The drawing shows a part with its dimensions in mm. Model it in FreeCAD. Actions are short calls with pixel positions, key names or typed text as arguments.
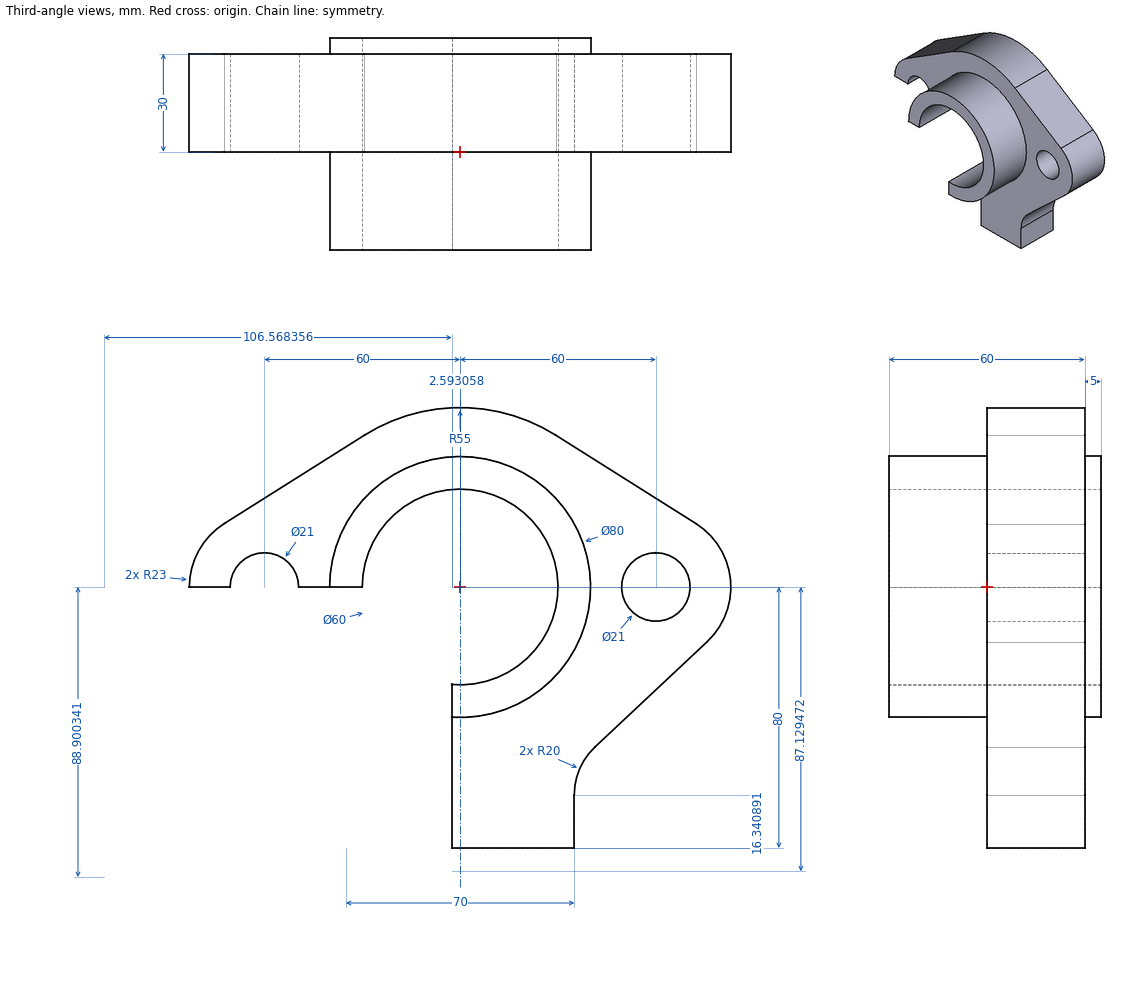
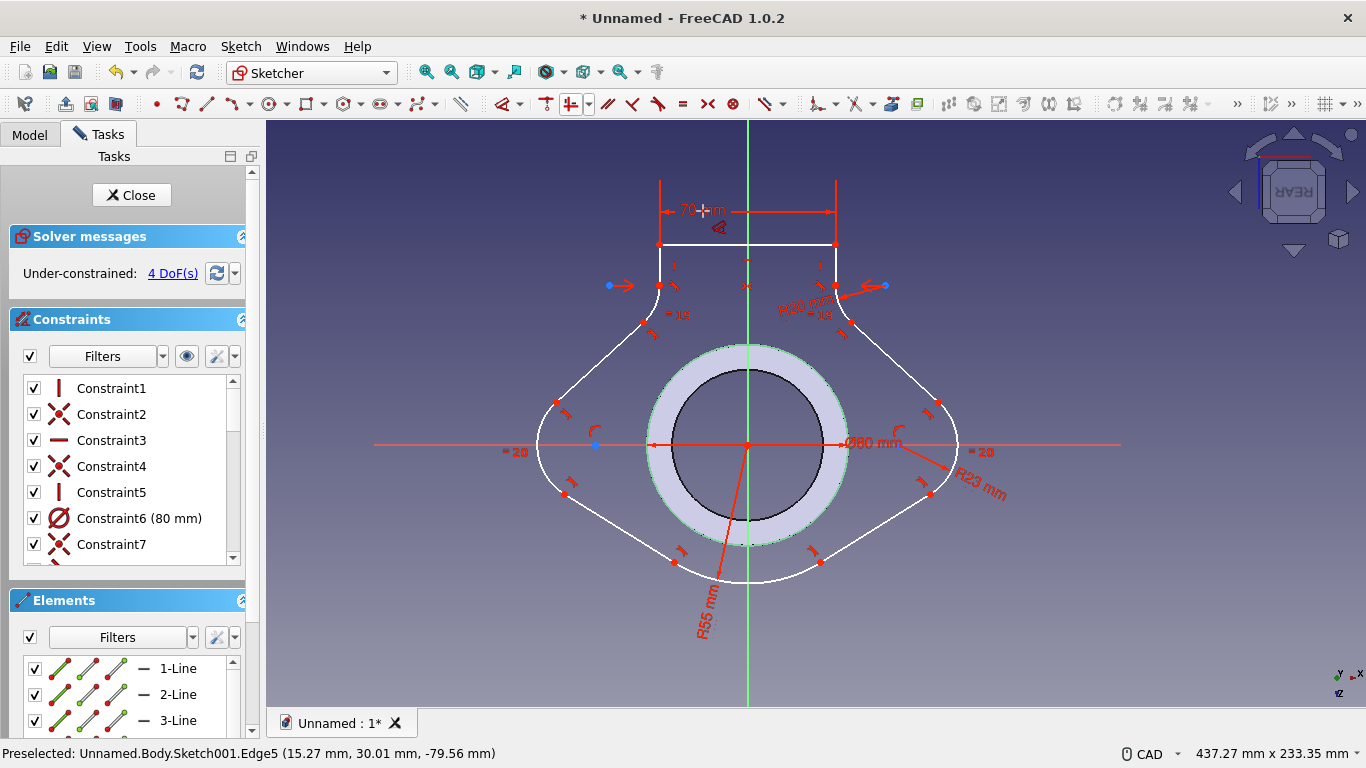
click(836, 245)
click(870, 391)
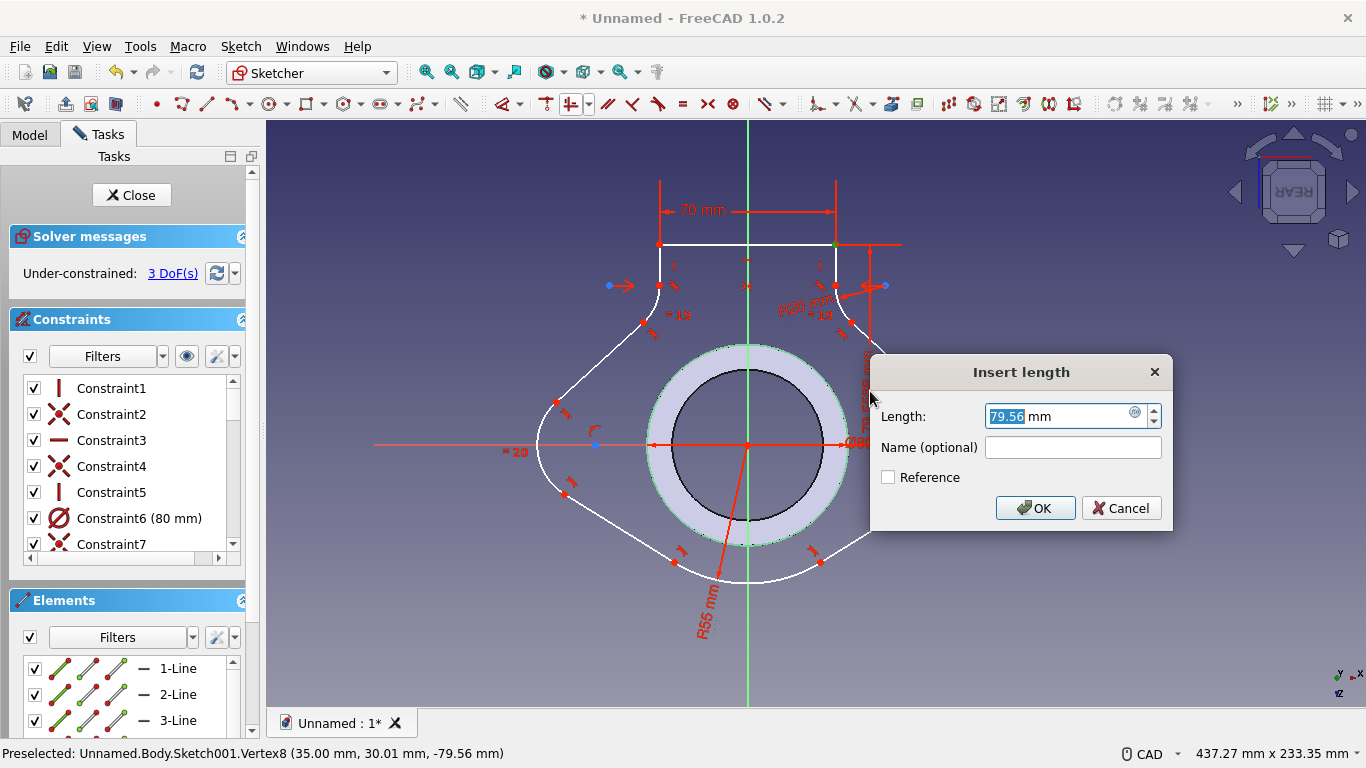
text(80)
key(Return)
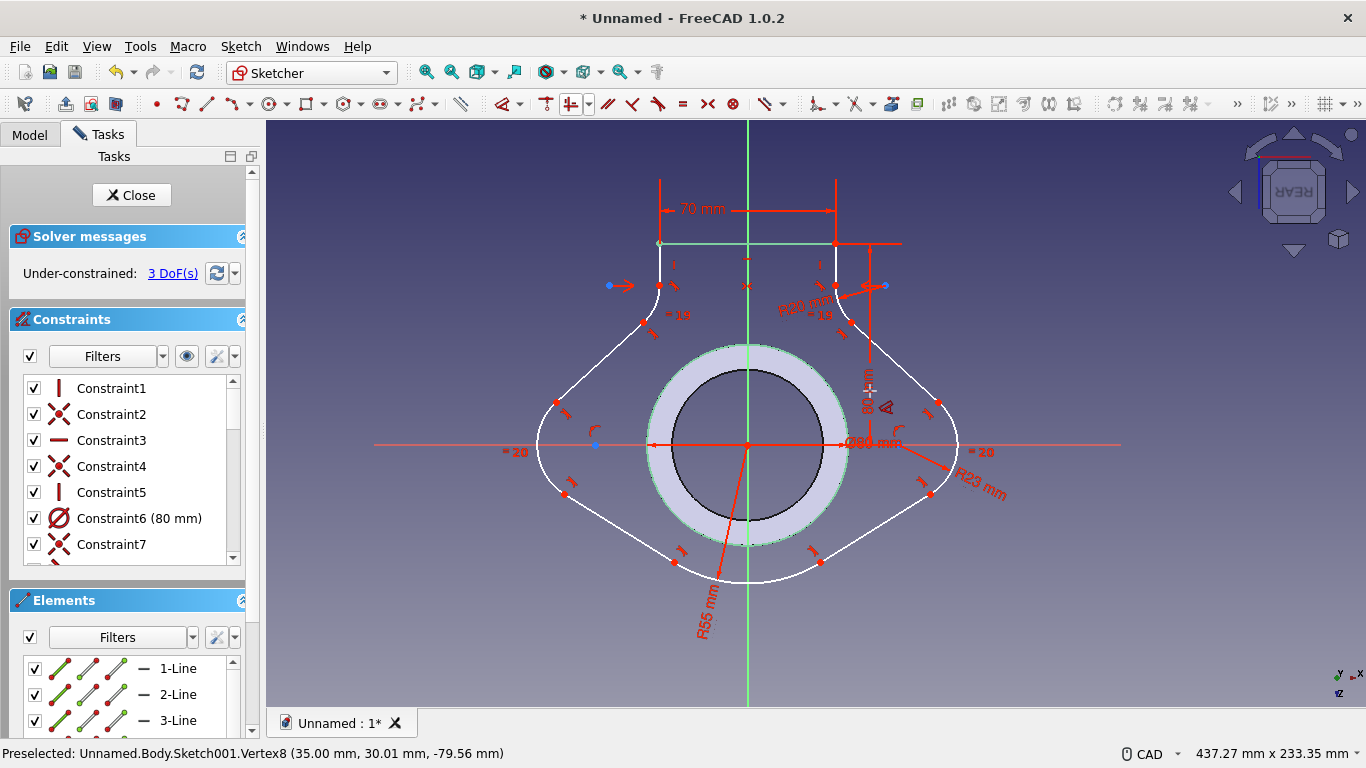
click(900, 445)
click(824, 479)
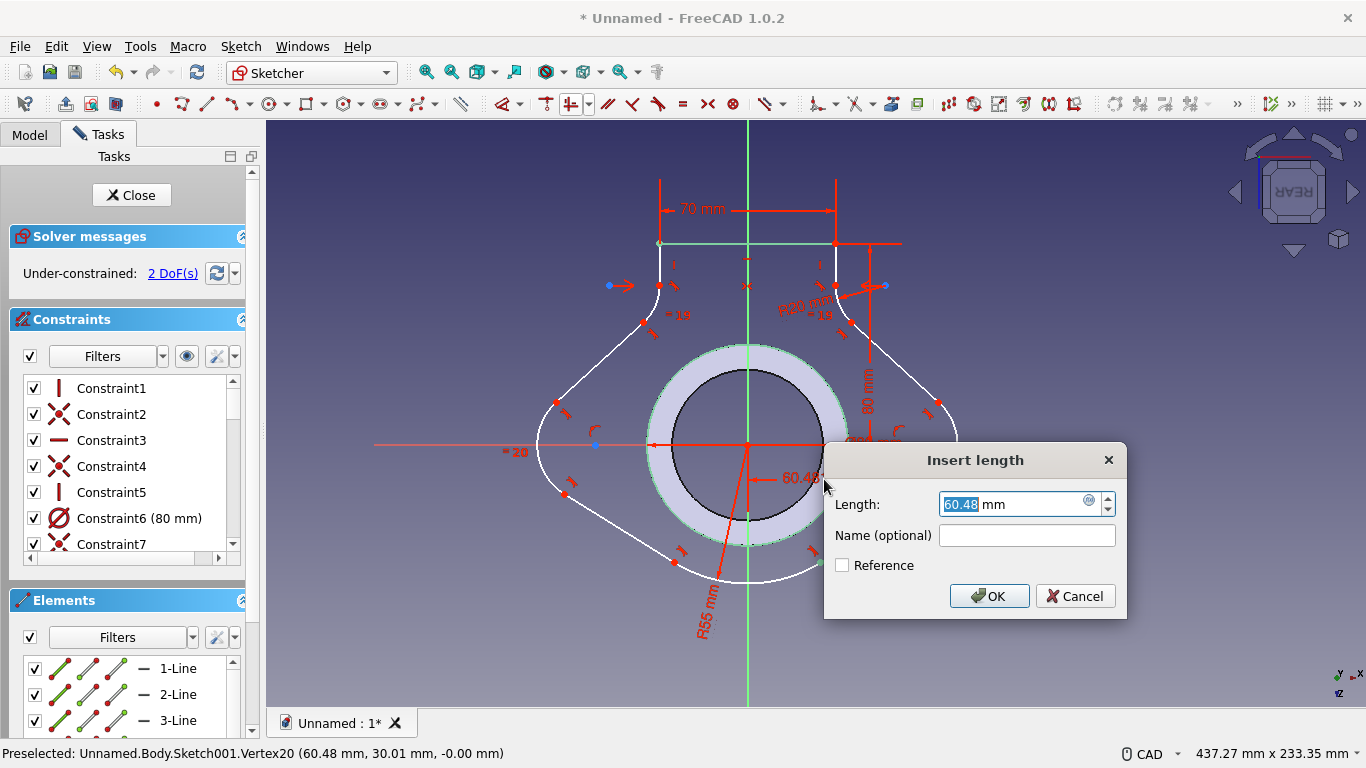
text(60)
key(Return)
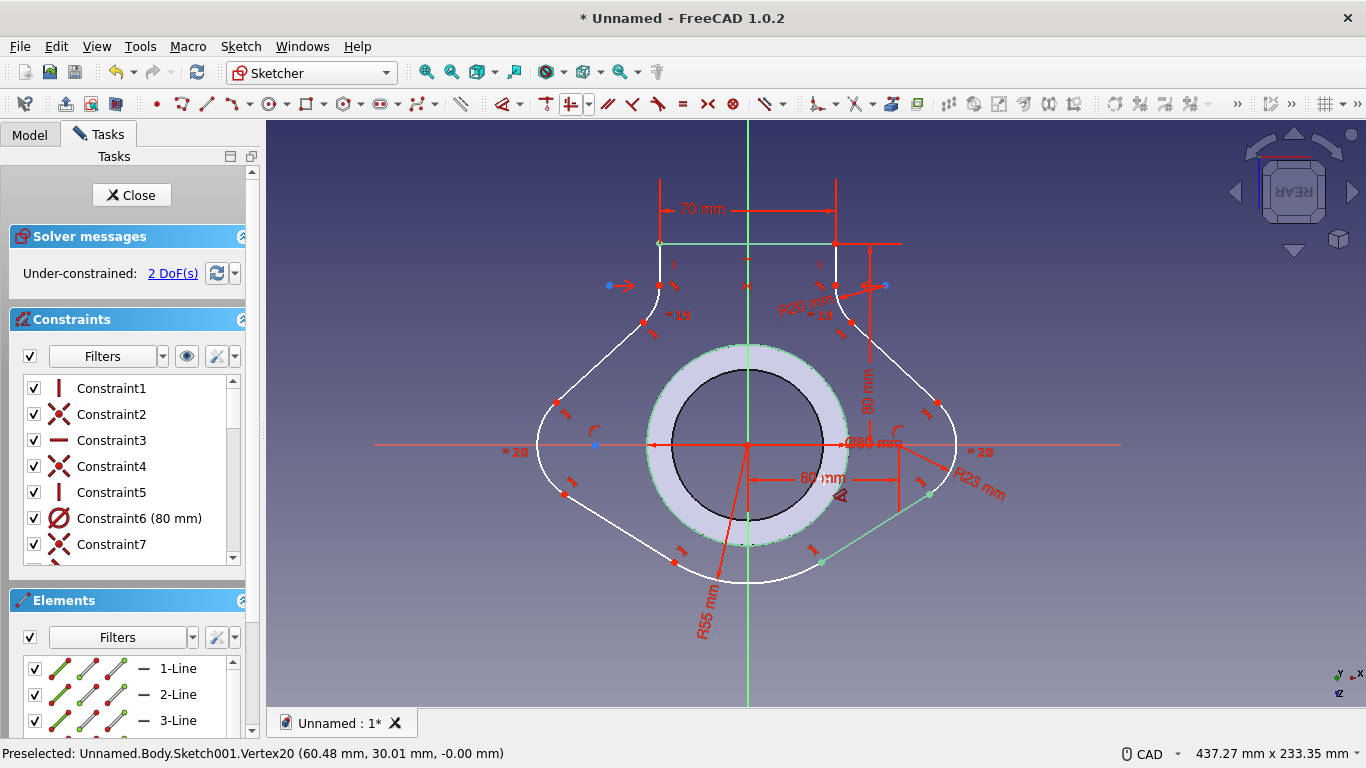
click(595, 445)
click(671, 479)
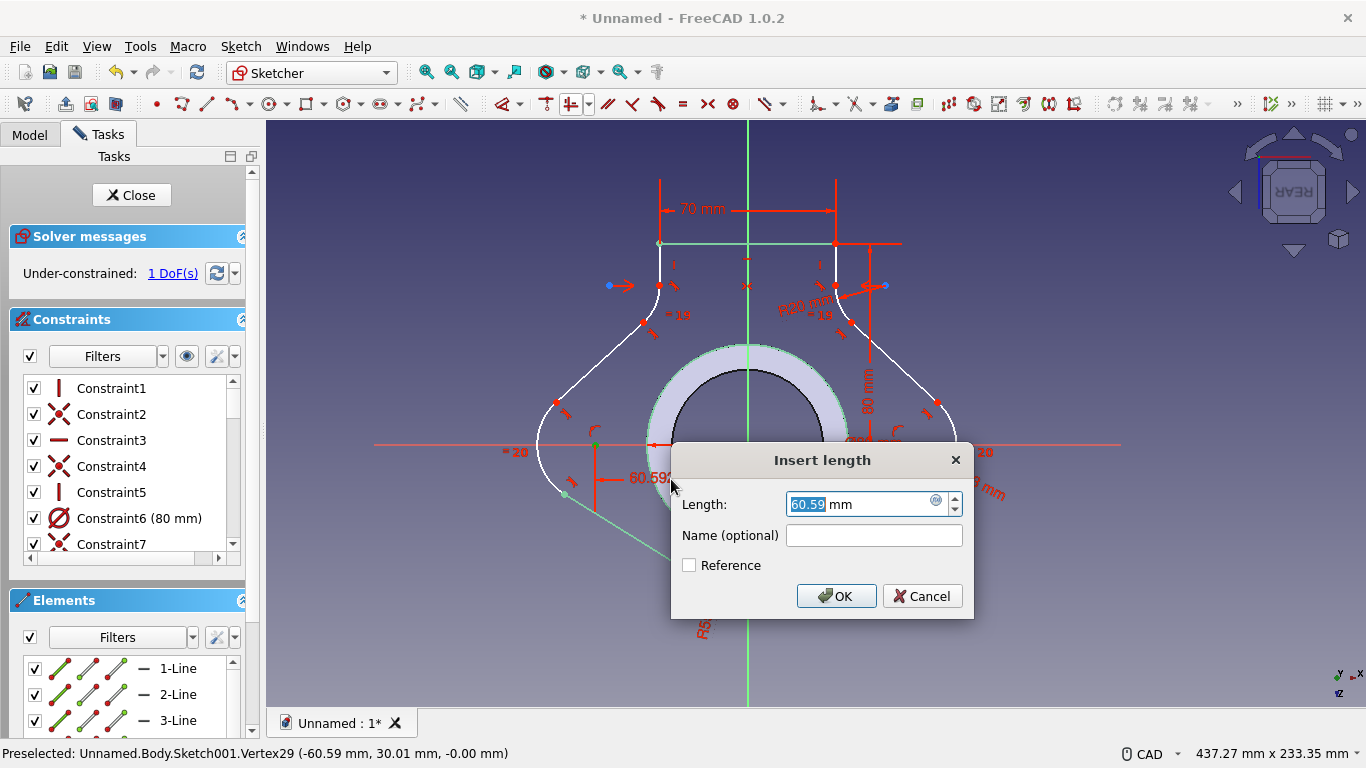
text(60)
key(Return)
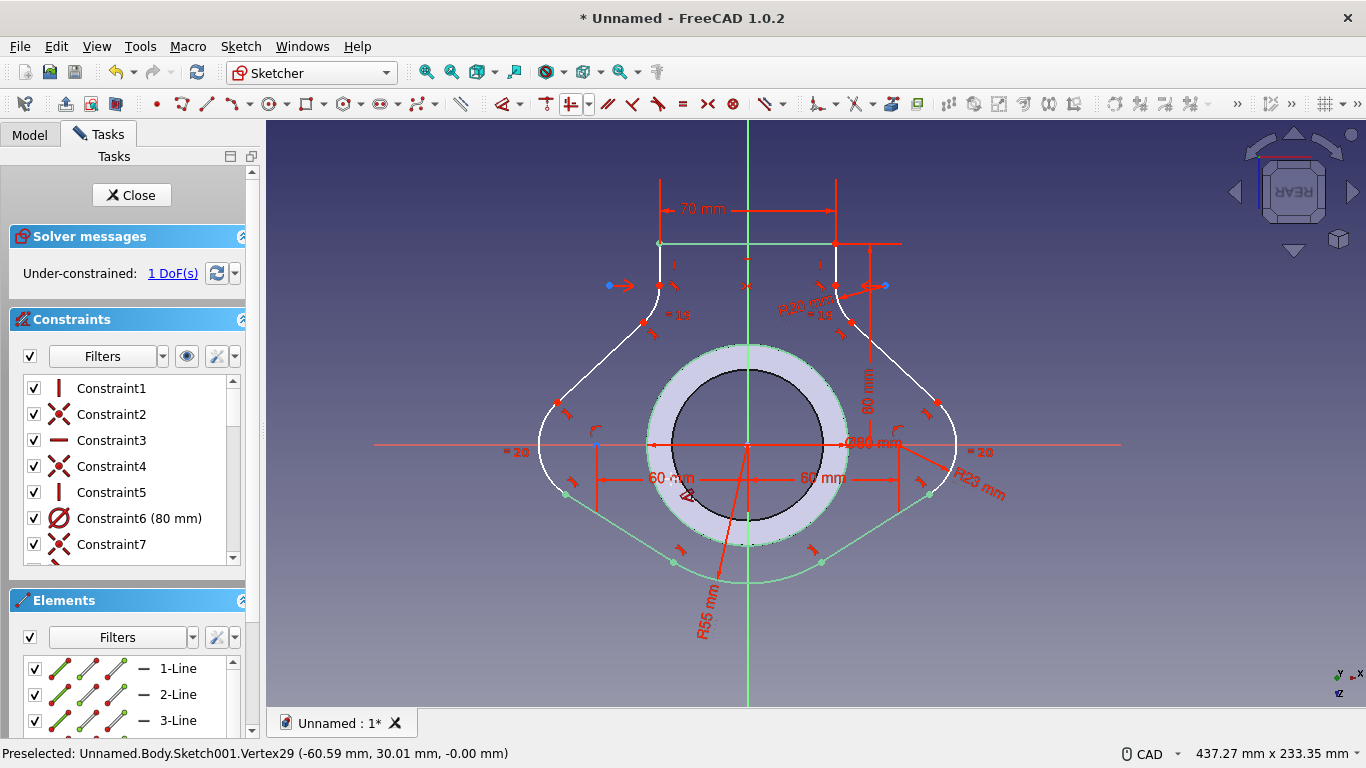
click(836, 273)
click(870, 265)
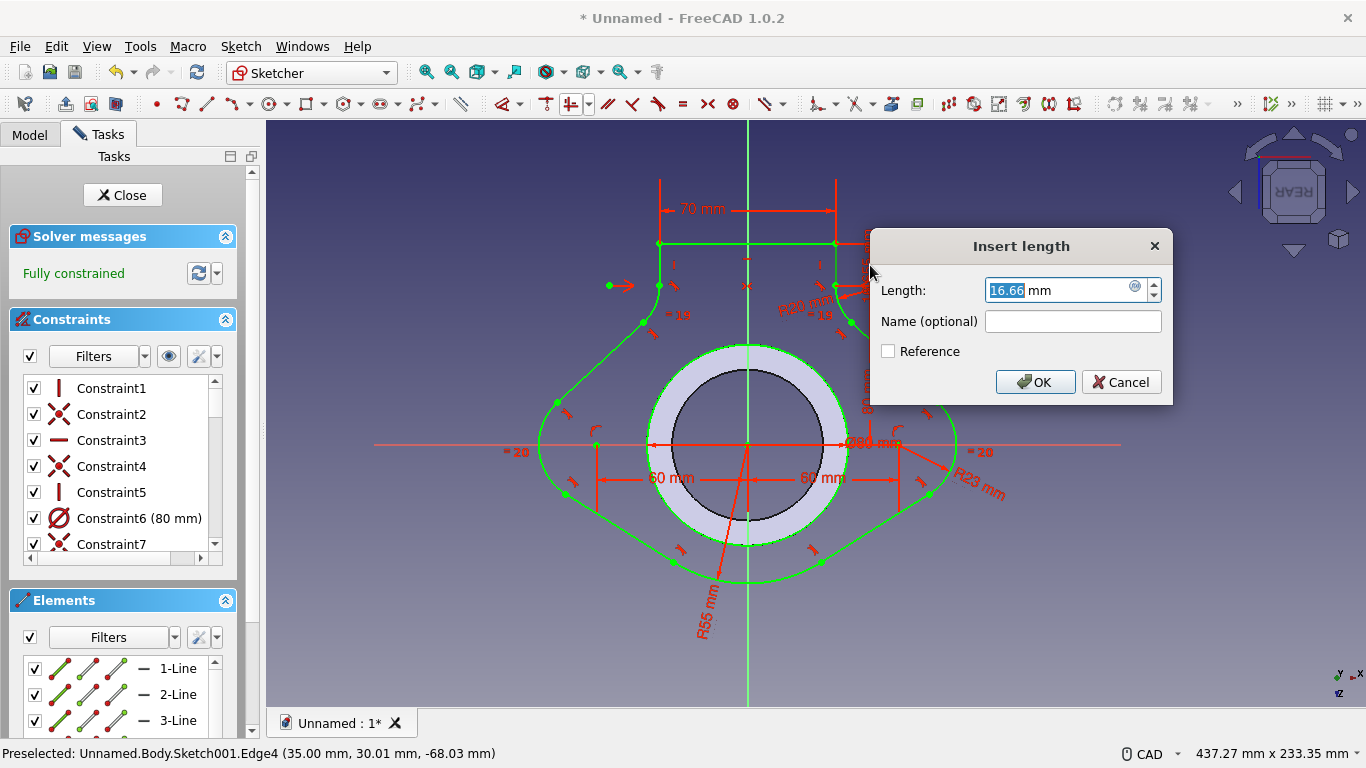
text(16.340891)
key(Return)
key(Escape)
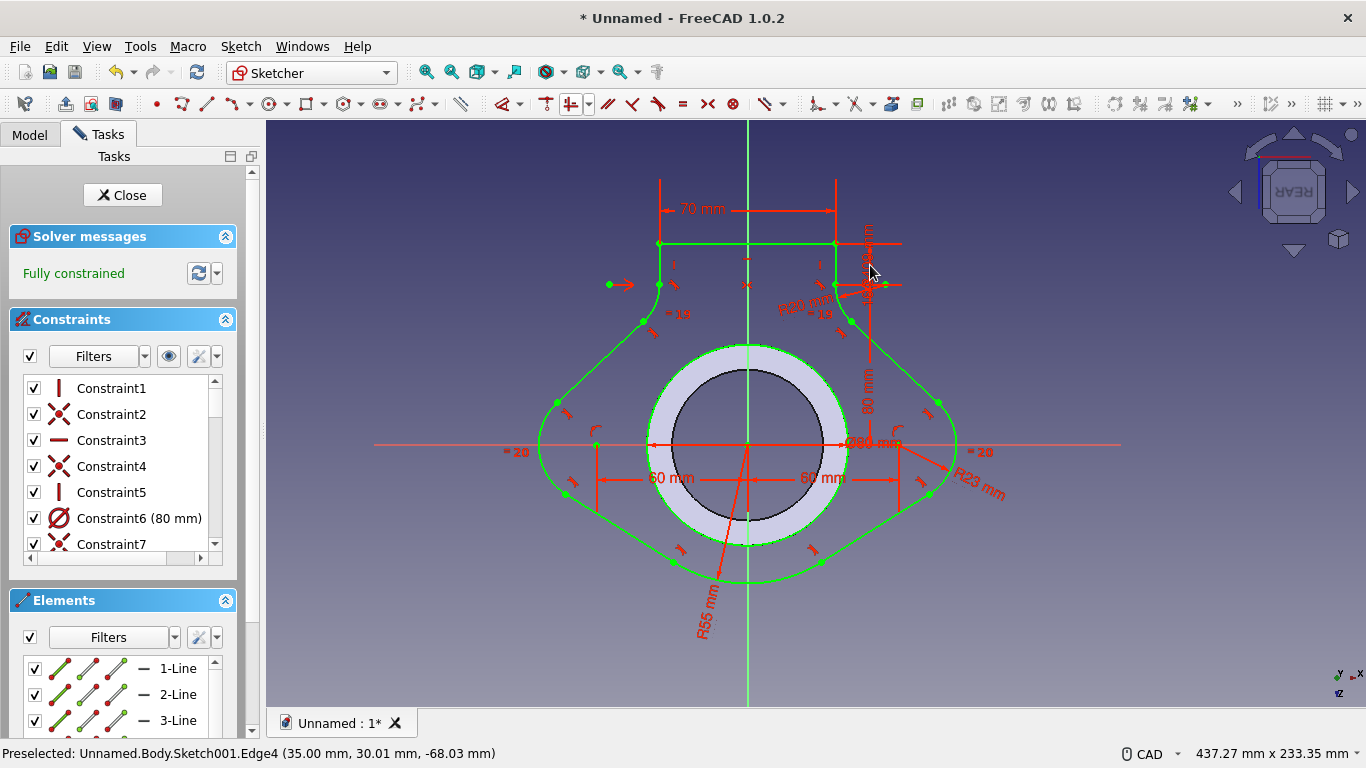
click(123, 195)